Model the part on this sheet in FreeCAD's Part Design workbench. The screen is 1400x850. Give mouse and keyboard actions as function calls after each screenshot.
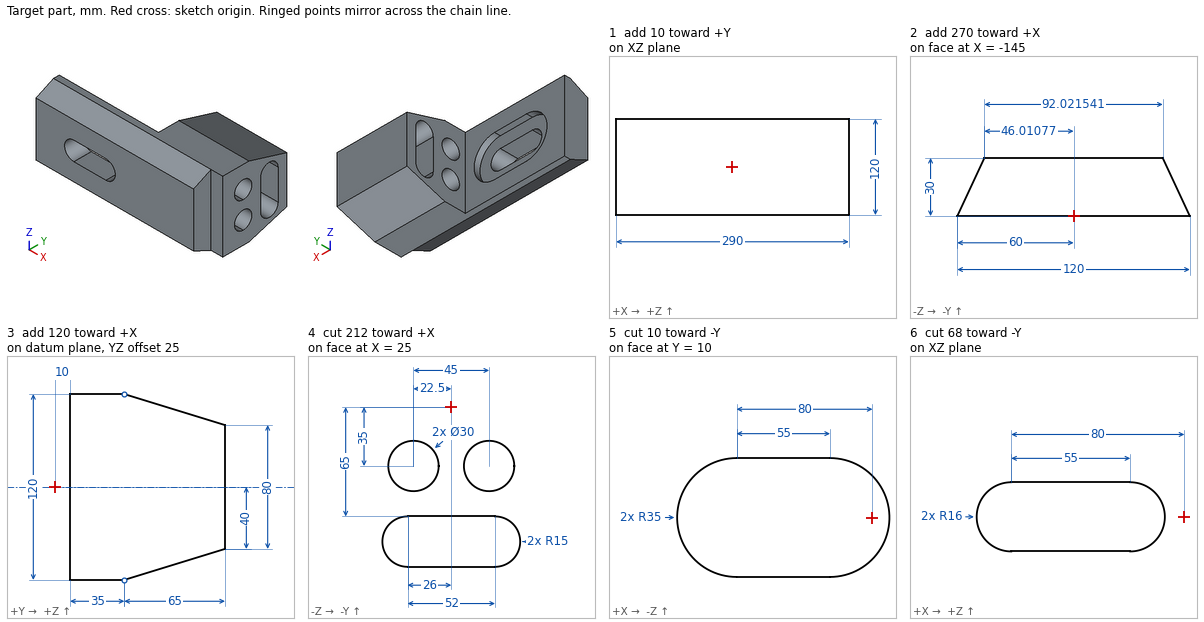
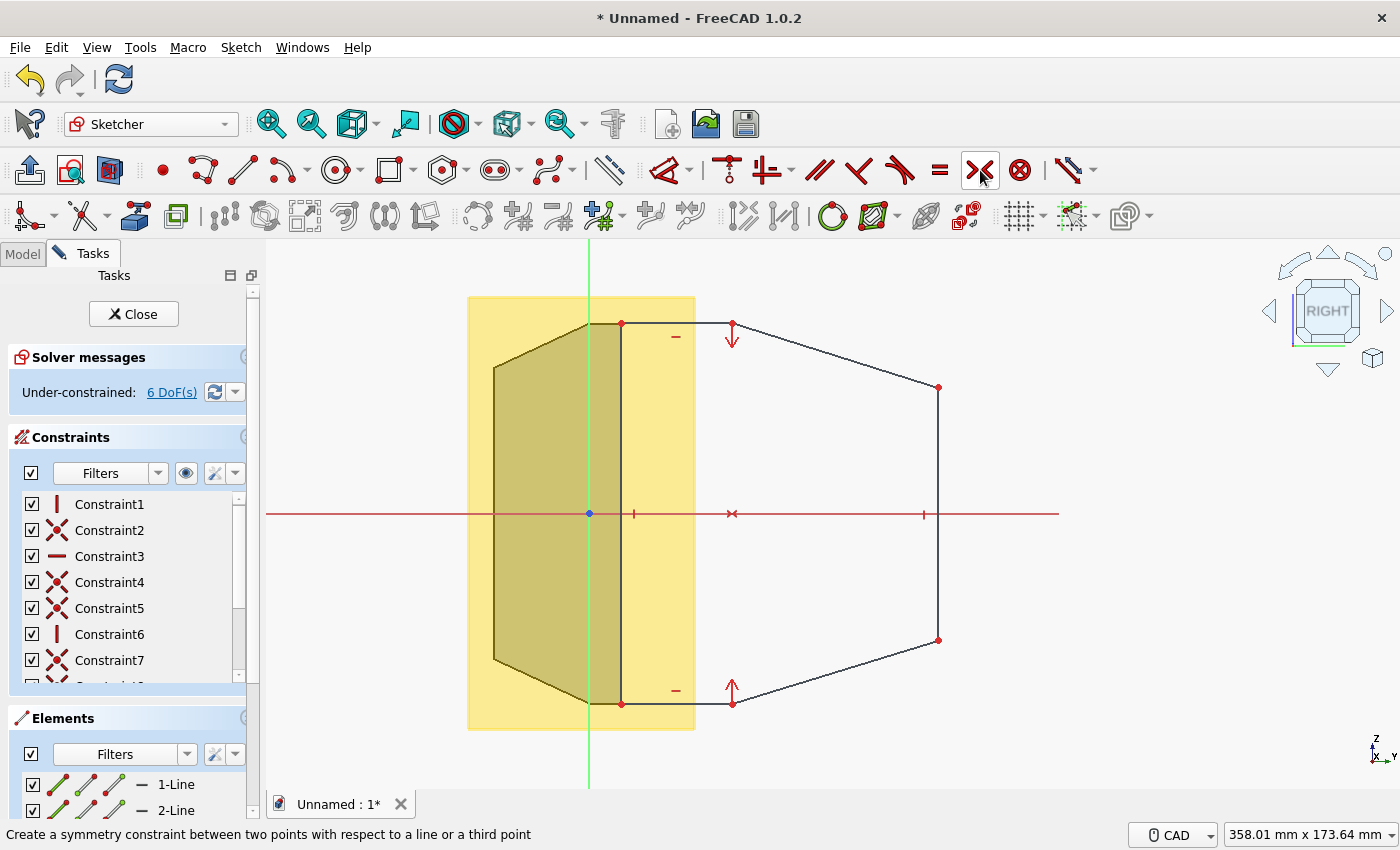
key(d)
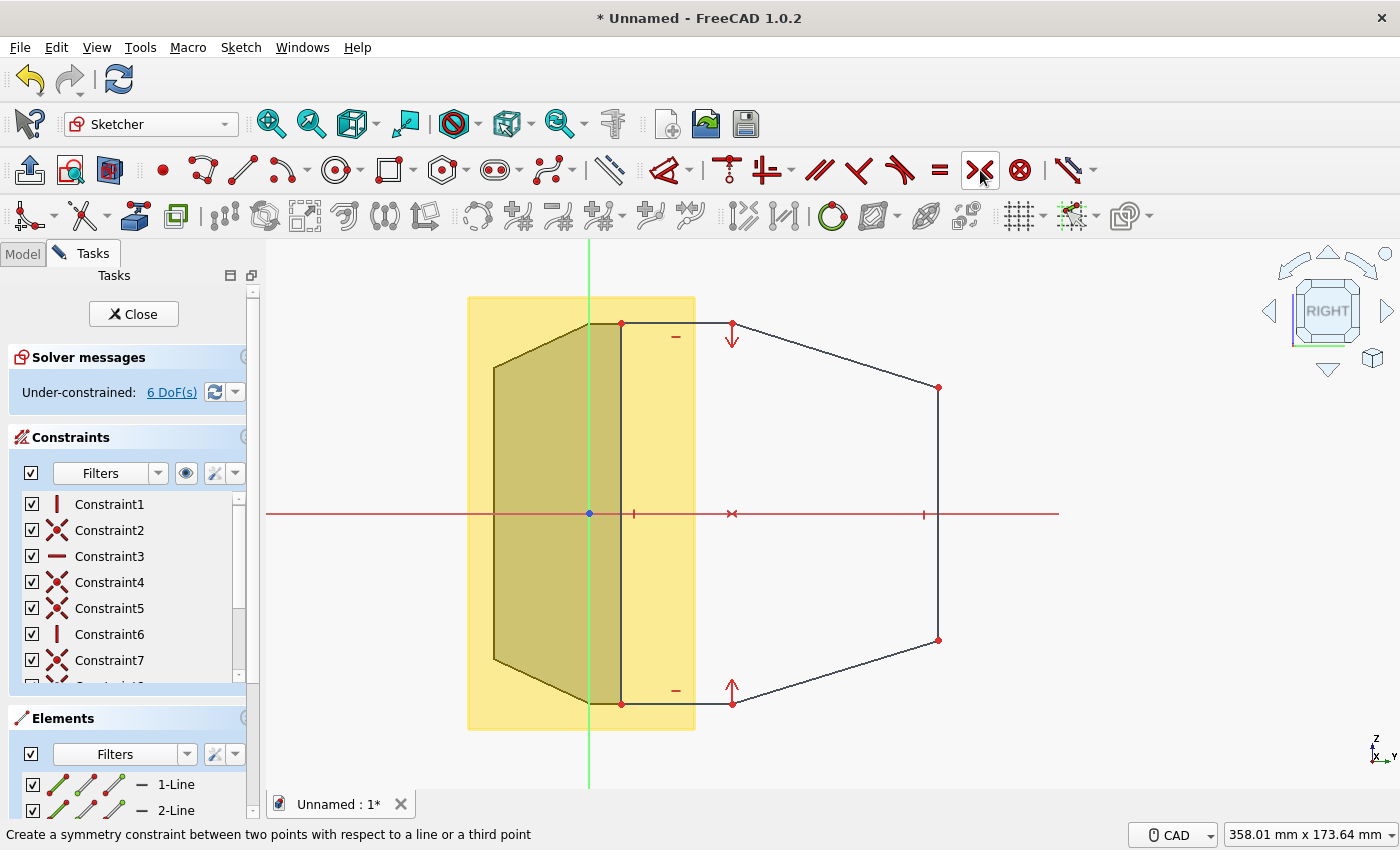
click(654, 704)
click(676, 738)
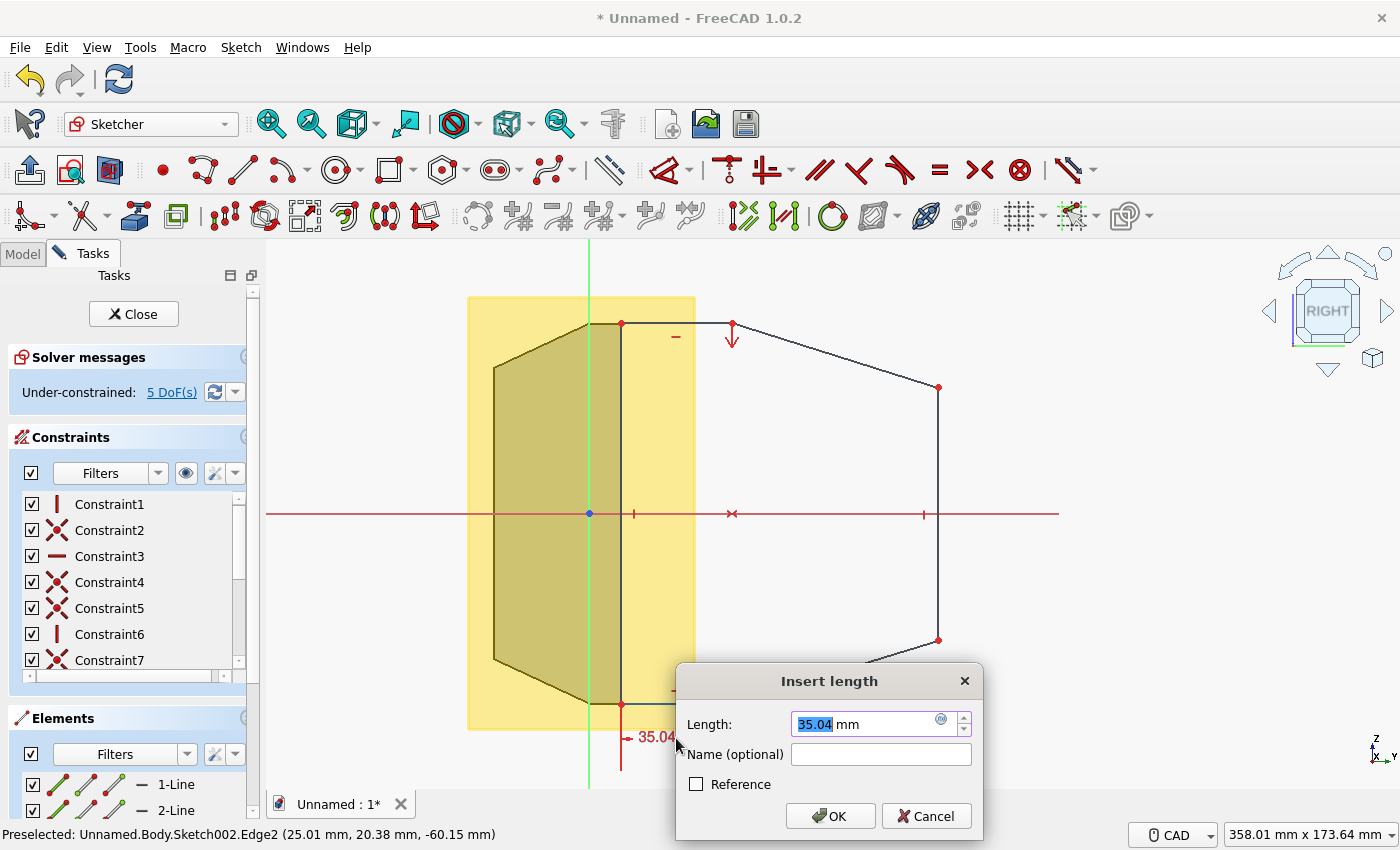
text(35)
key(Return)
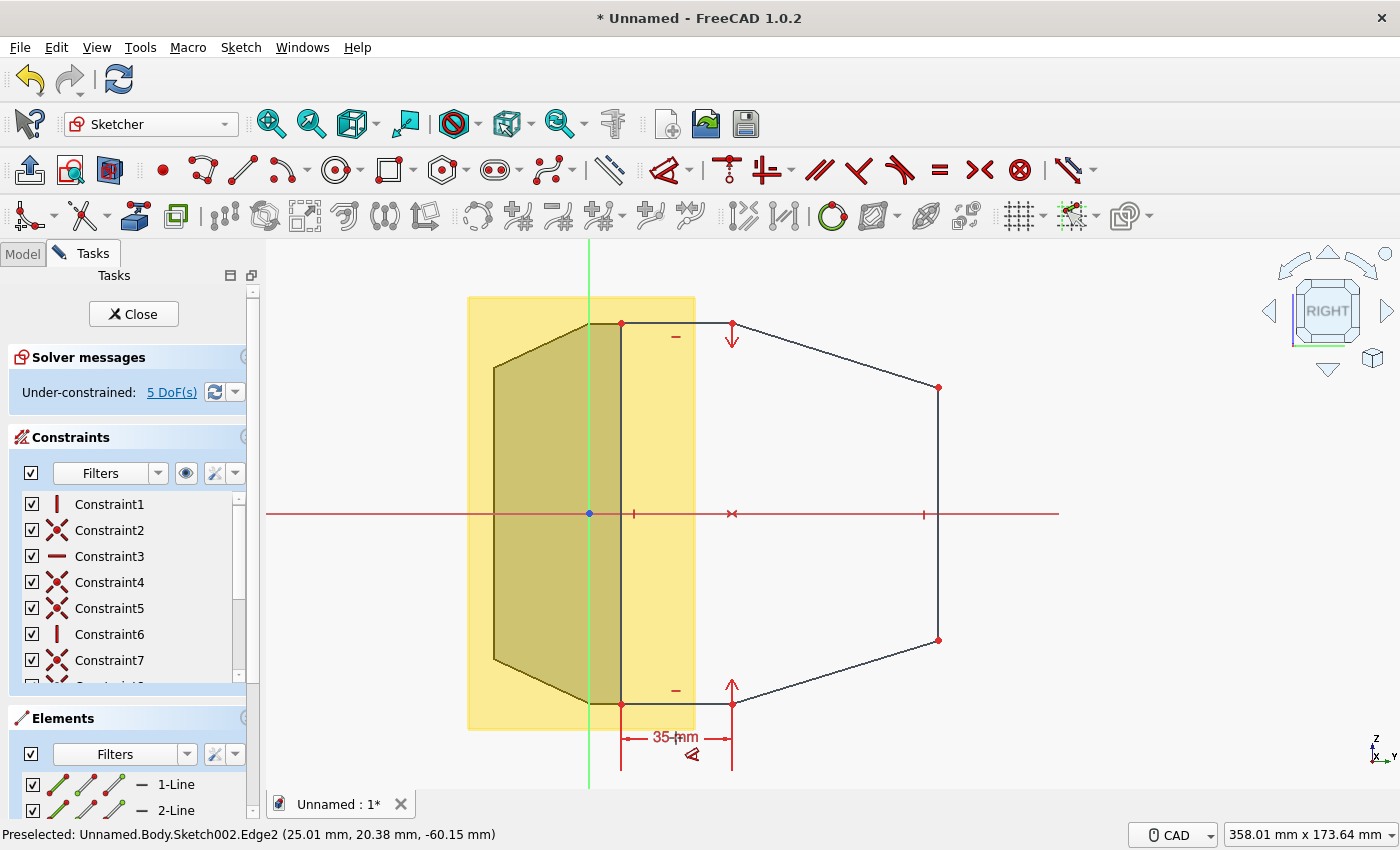
click(938, 565)
click(972, 456)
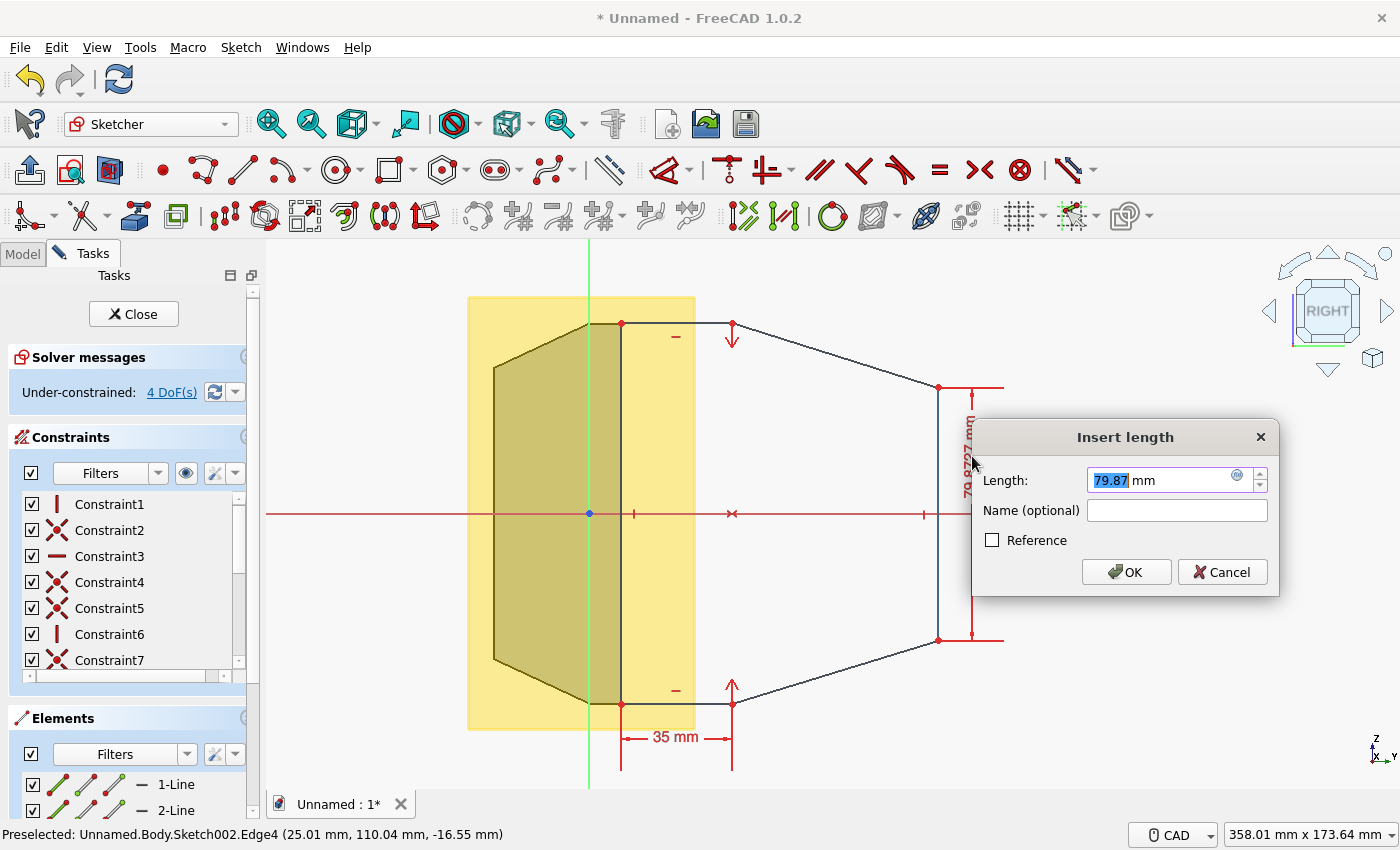
text(80)
key(Return)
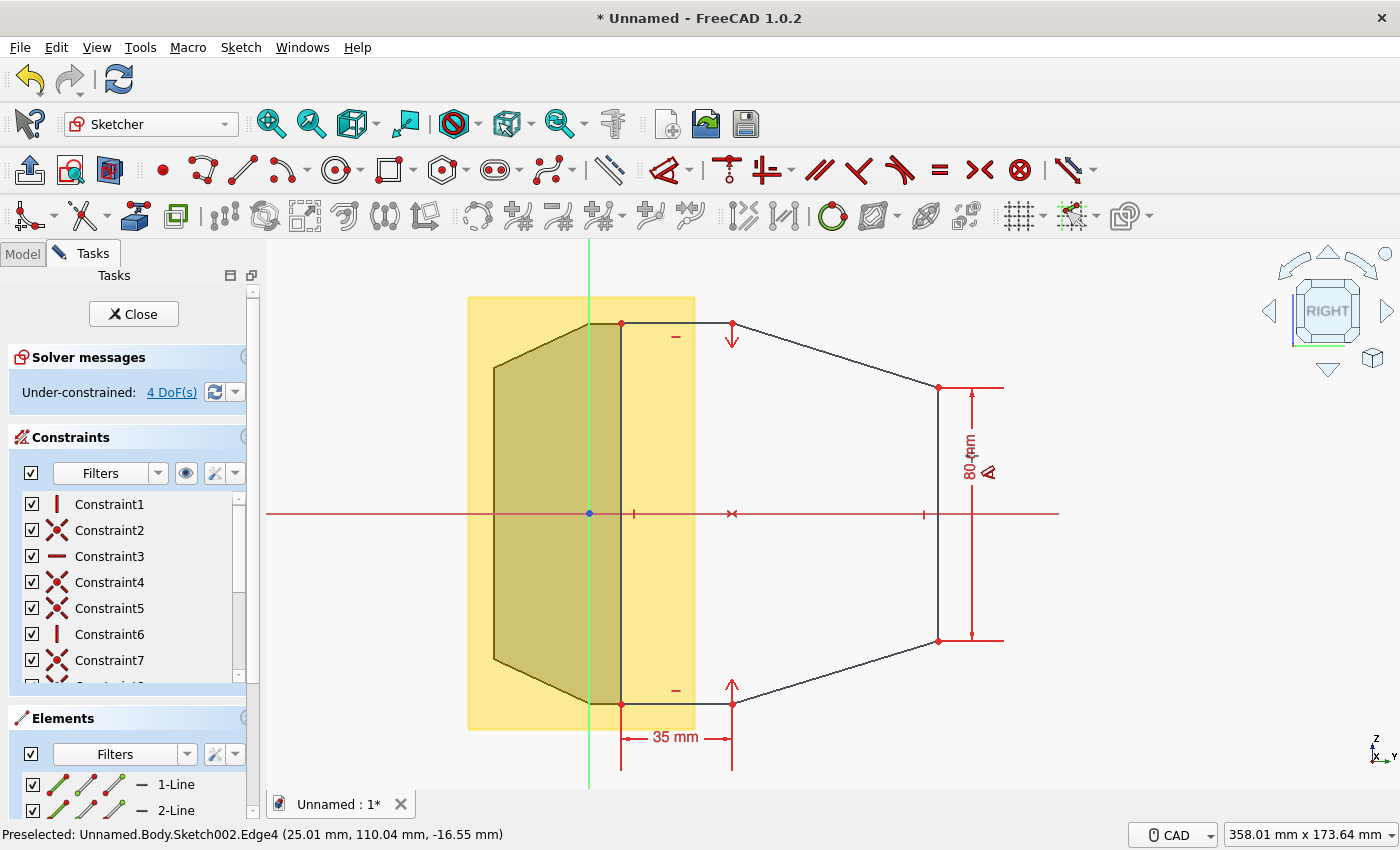
click(621, 437)
click(655, 426)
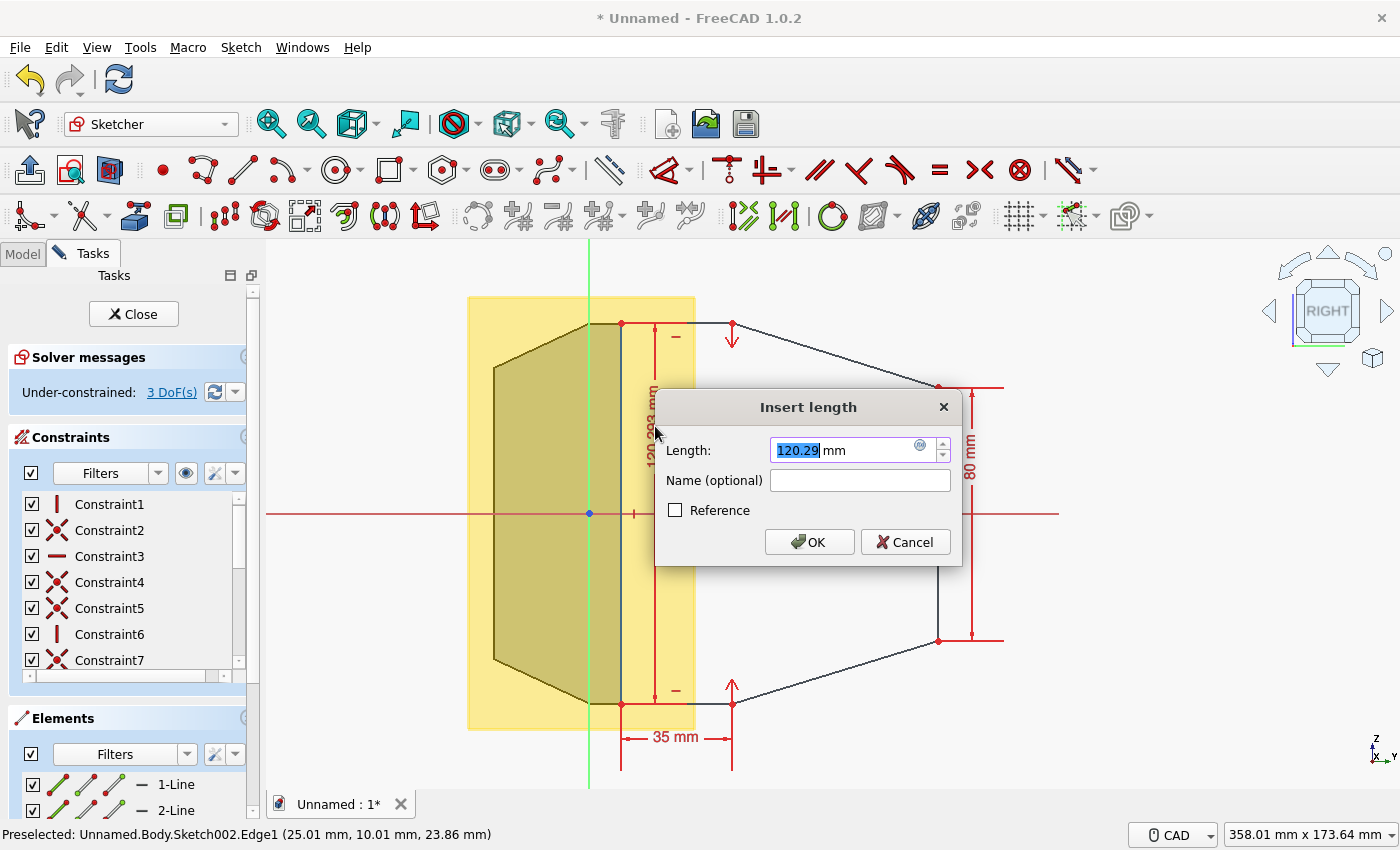
text(120)
key(Return)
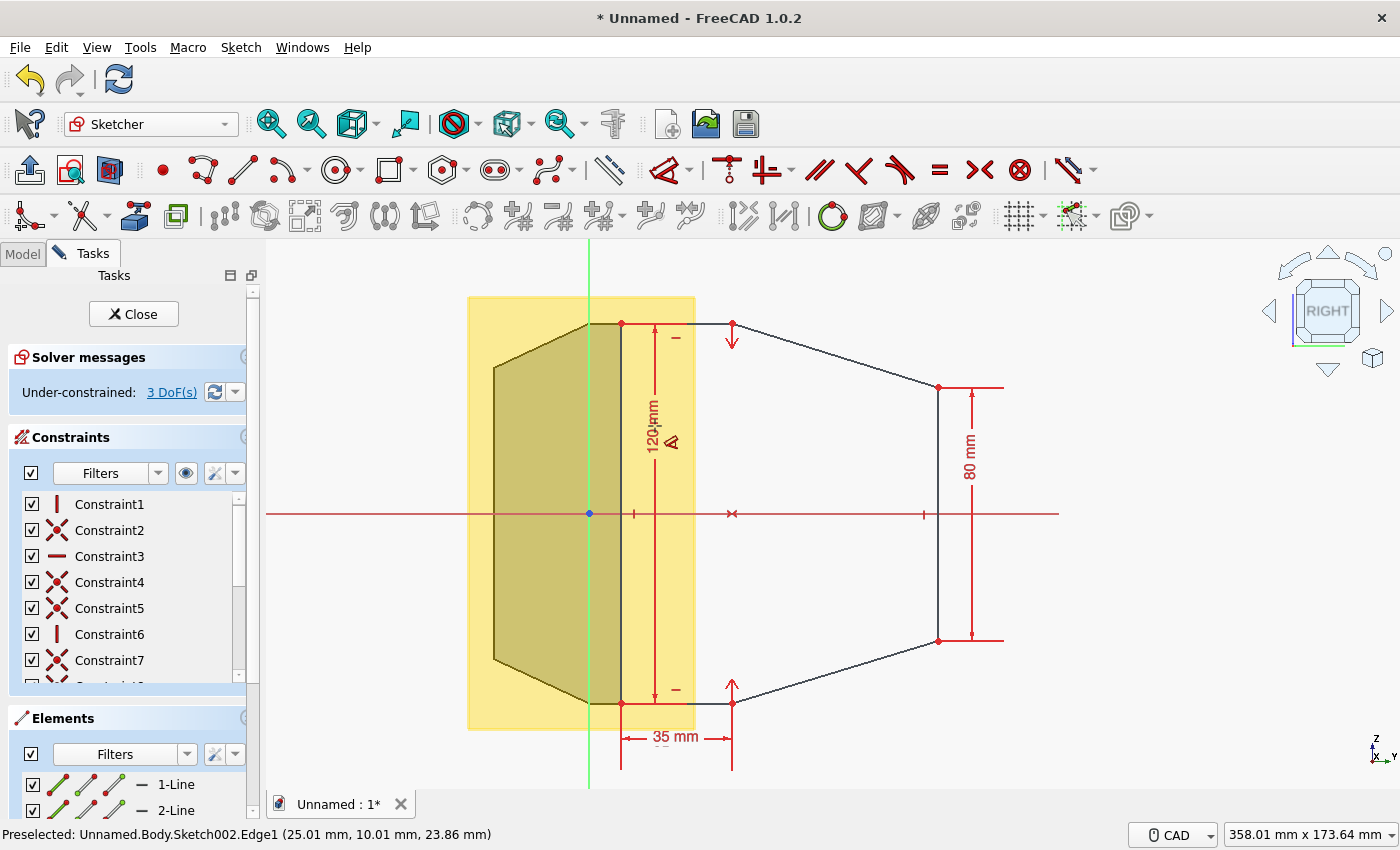
scroll(621, 324, up, 2)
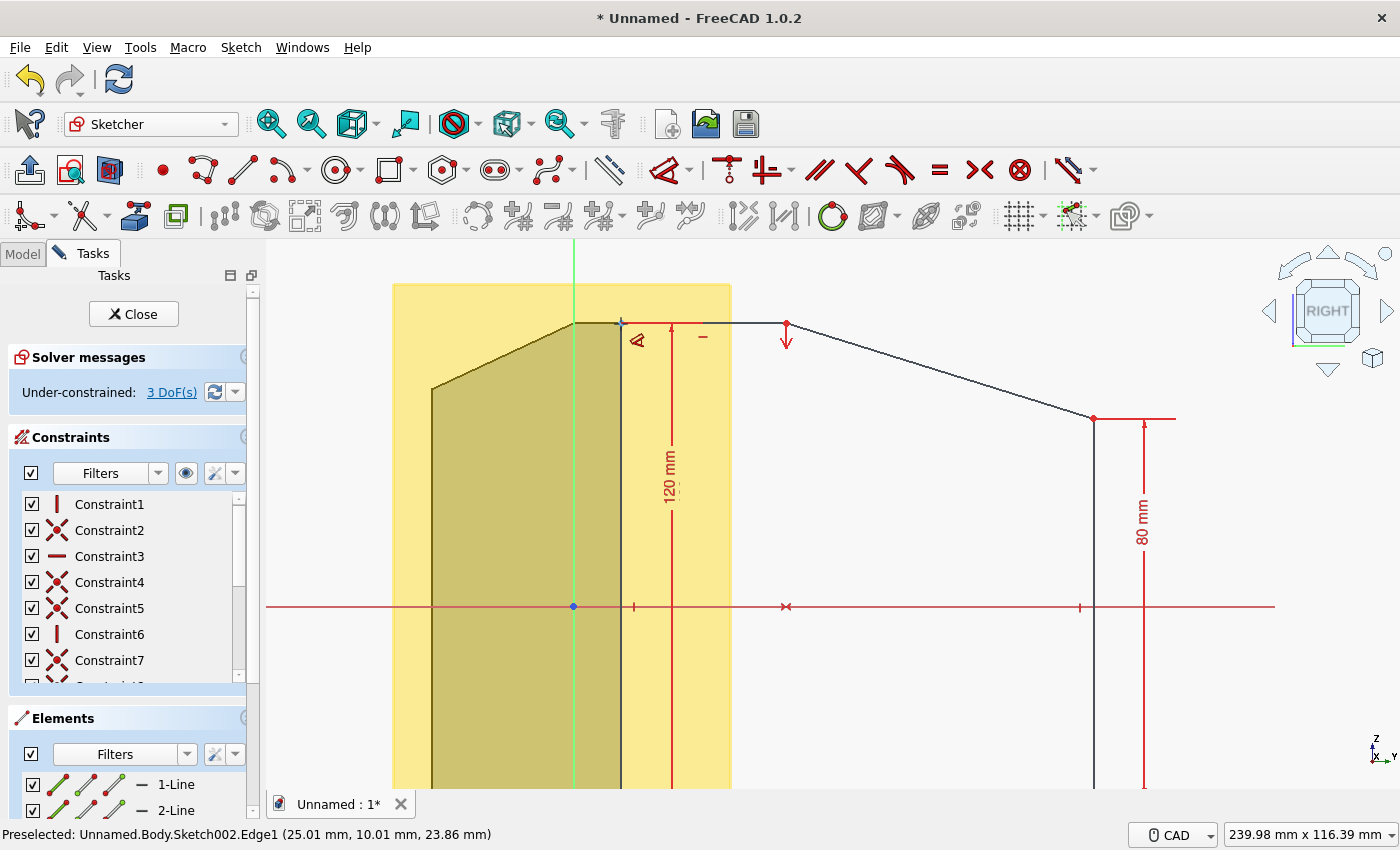
click(621, 323)
click(597, 289)